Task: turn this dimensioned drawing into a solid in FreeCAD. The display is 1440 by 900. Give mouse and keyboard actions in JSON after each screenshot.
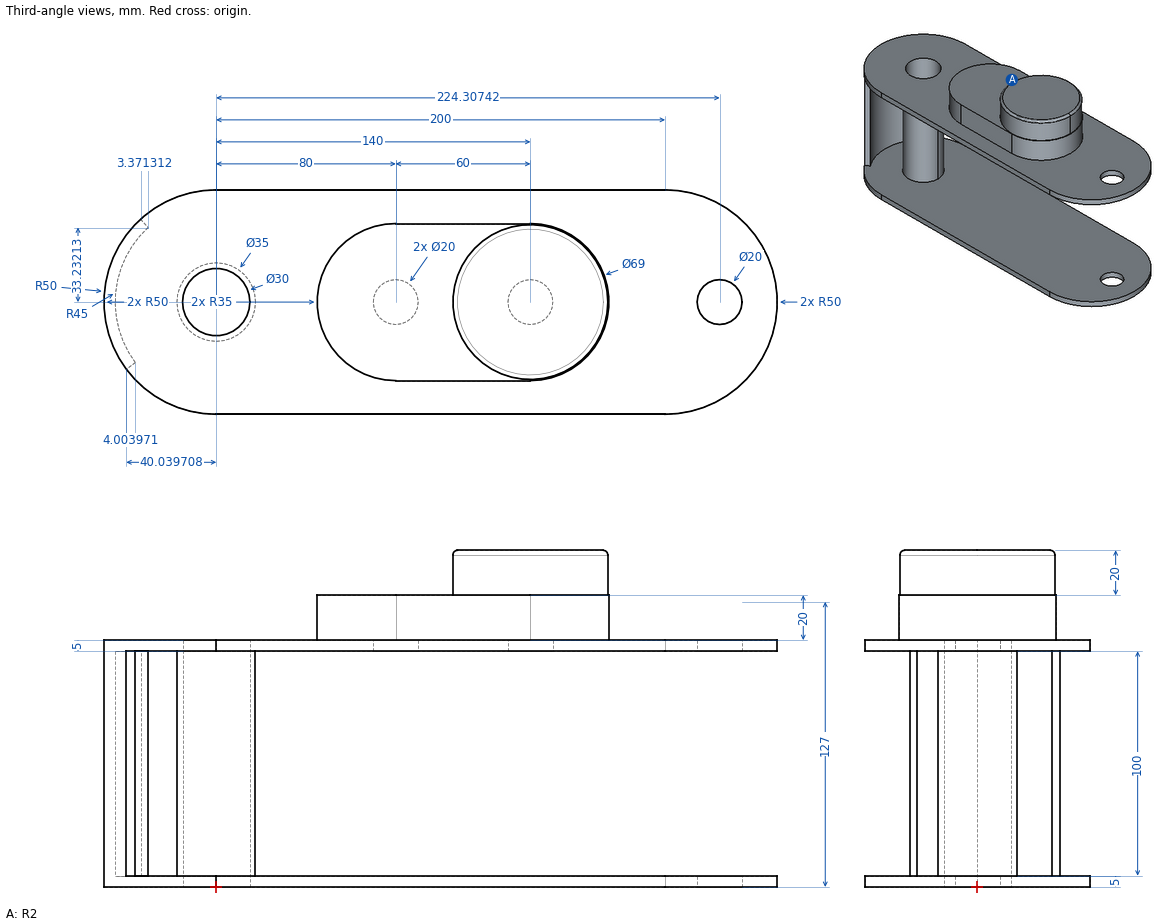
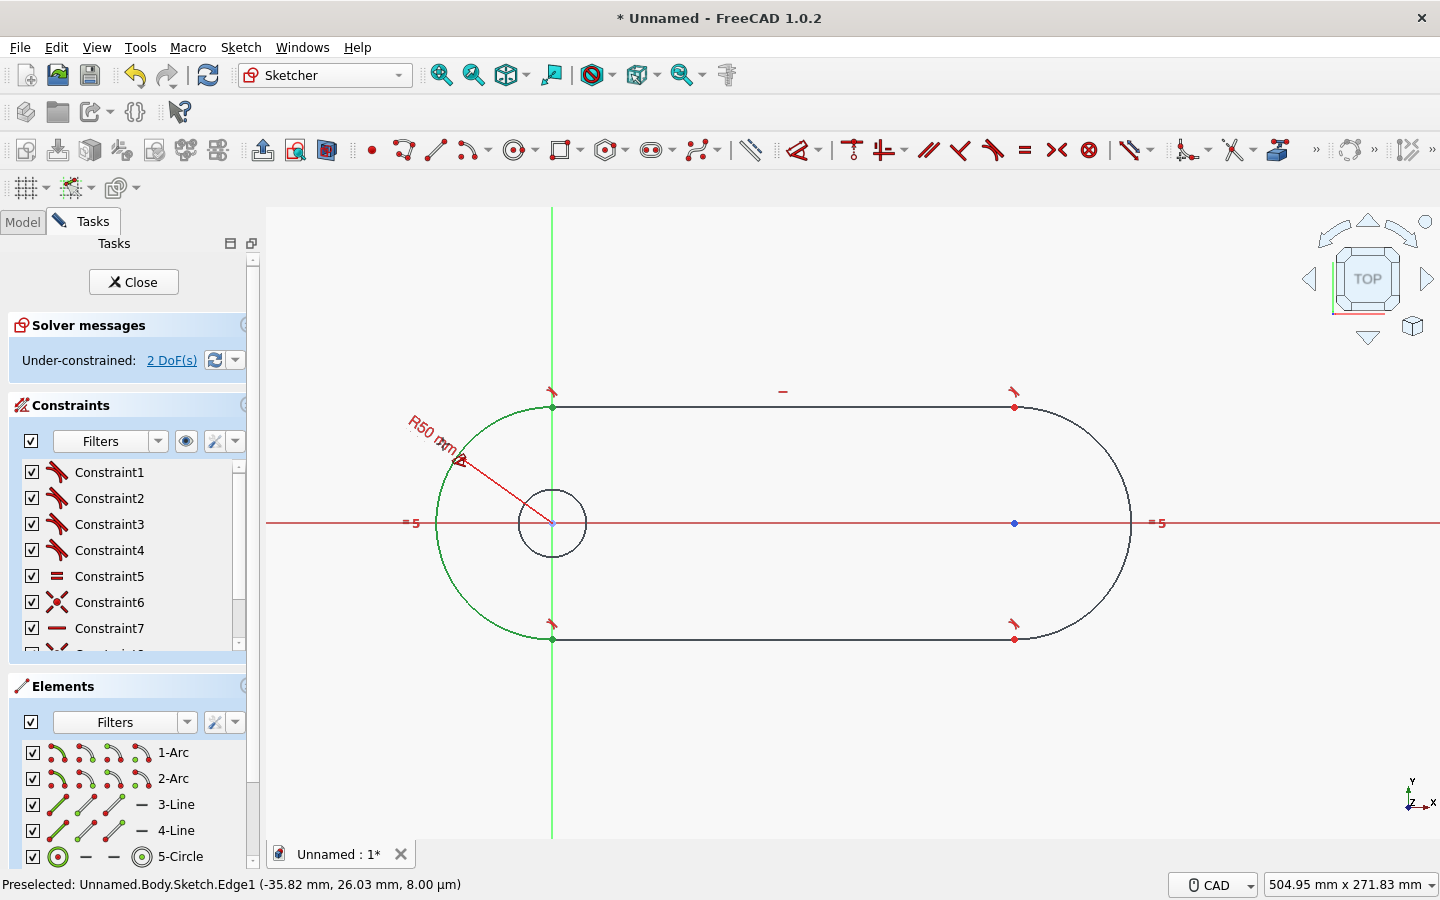
{"action": "left_click", "coordinate": [576, 499]}
{"action": "left_click", "coordinate": [598, 476]}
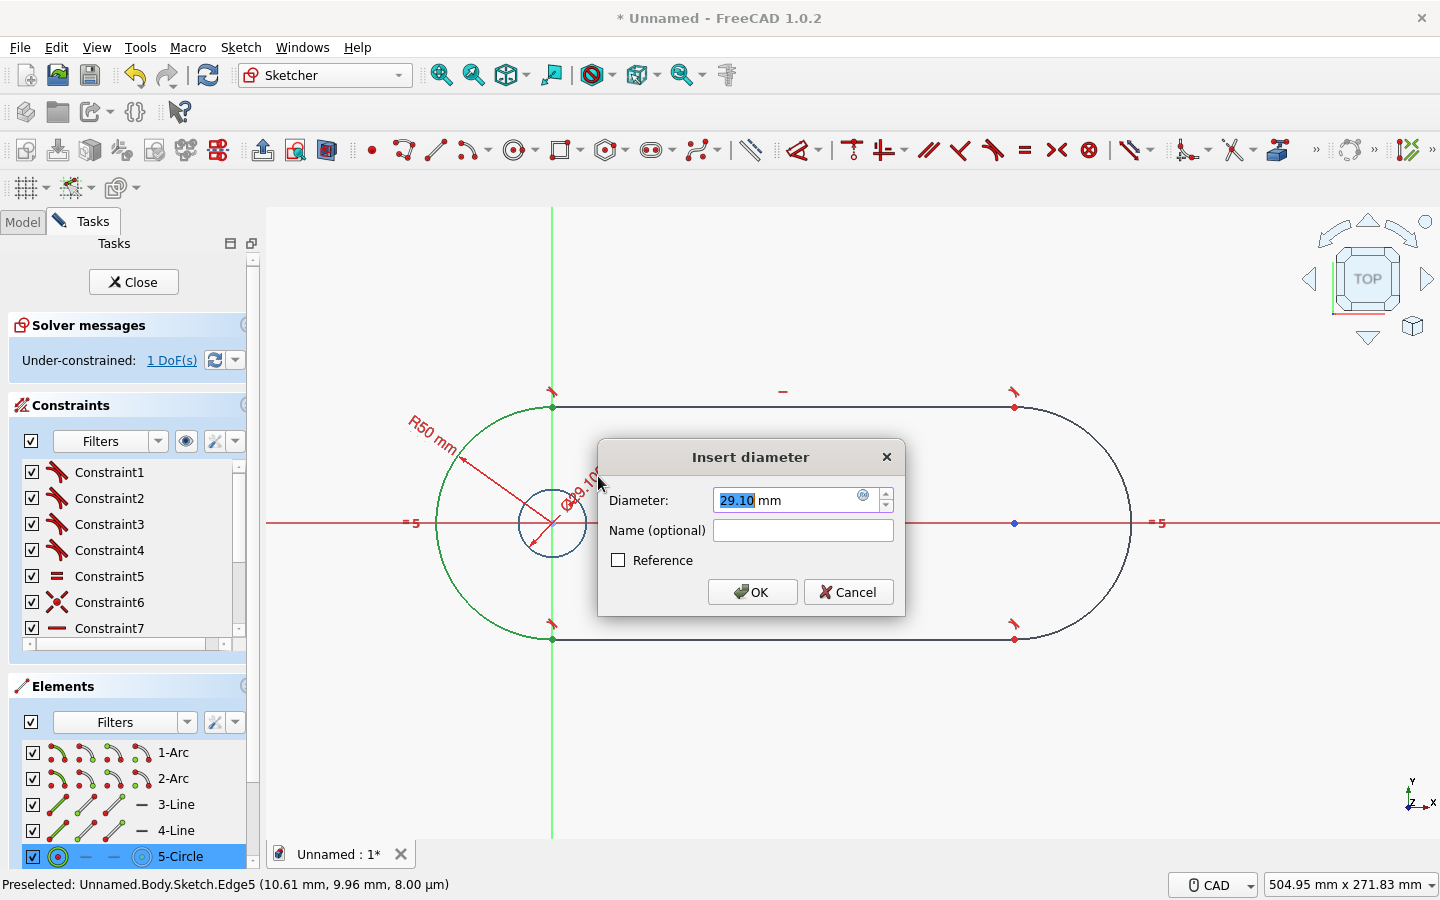
{"action": "type", "text": "30"}
{"action": "key", "text": "Return"}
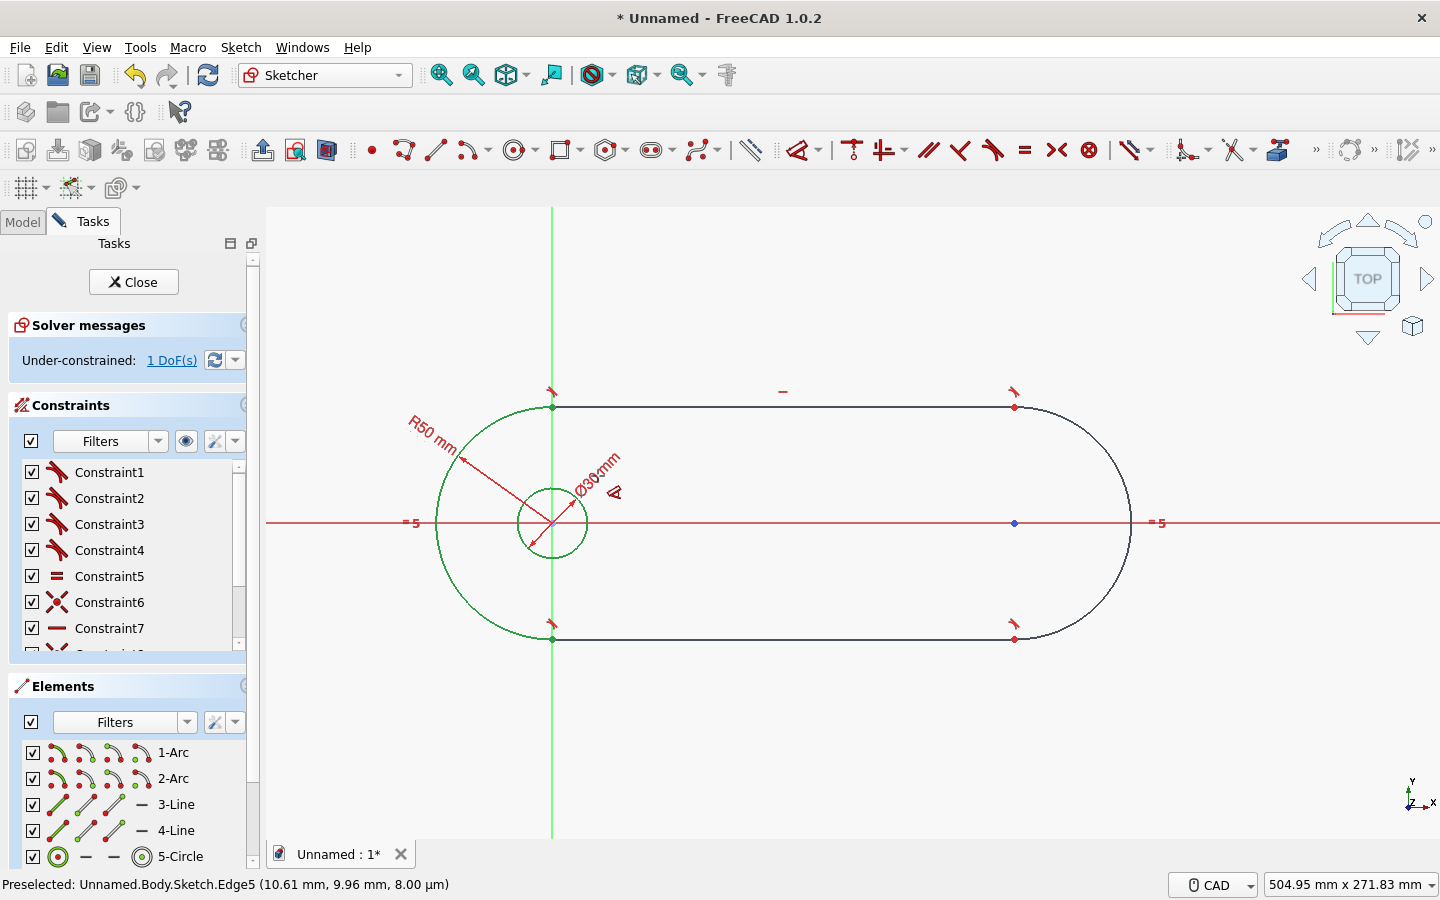
{"action": "left_click", "coordinate": [691, 407]}
{"action": "left_click", "coordinate": [784, 373]}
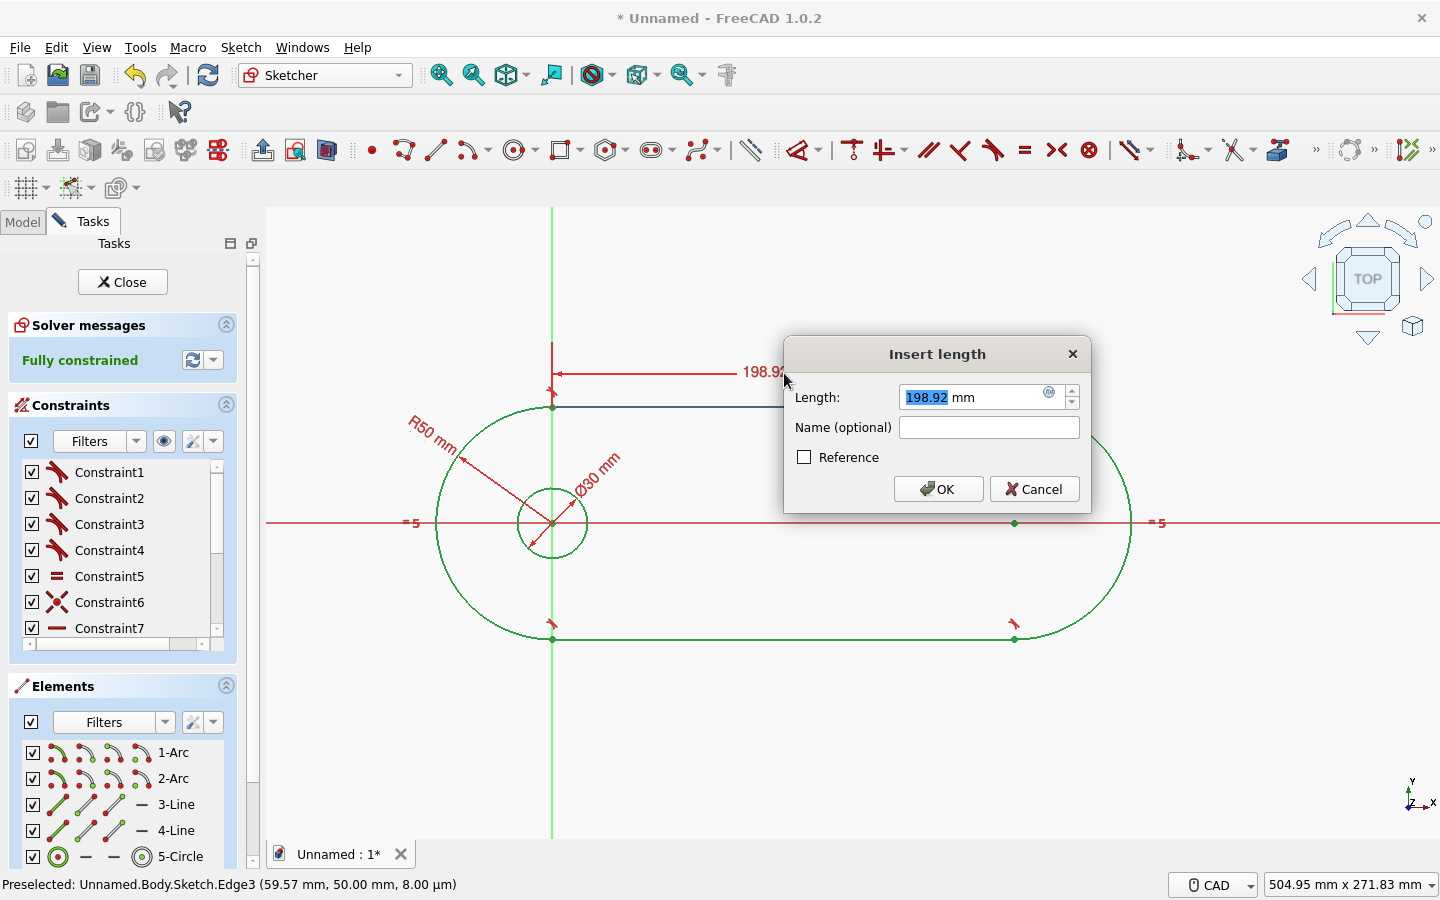
{"action": "type", "text": "200"}
{"action": "key", "text": "Return"}
{"action": "key", "text": "Escape"}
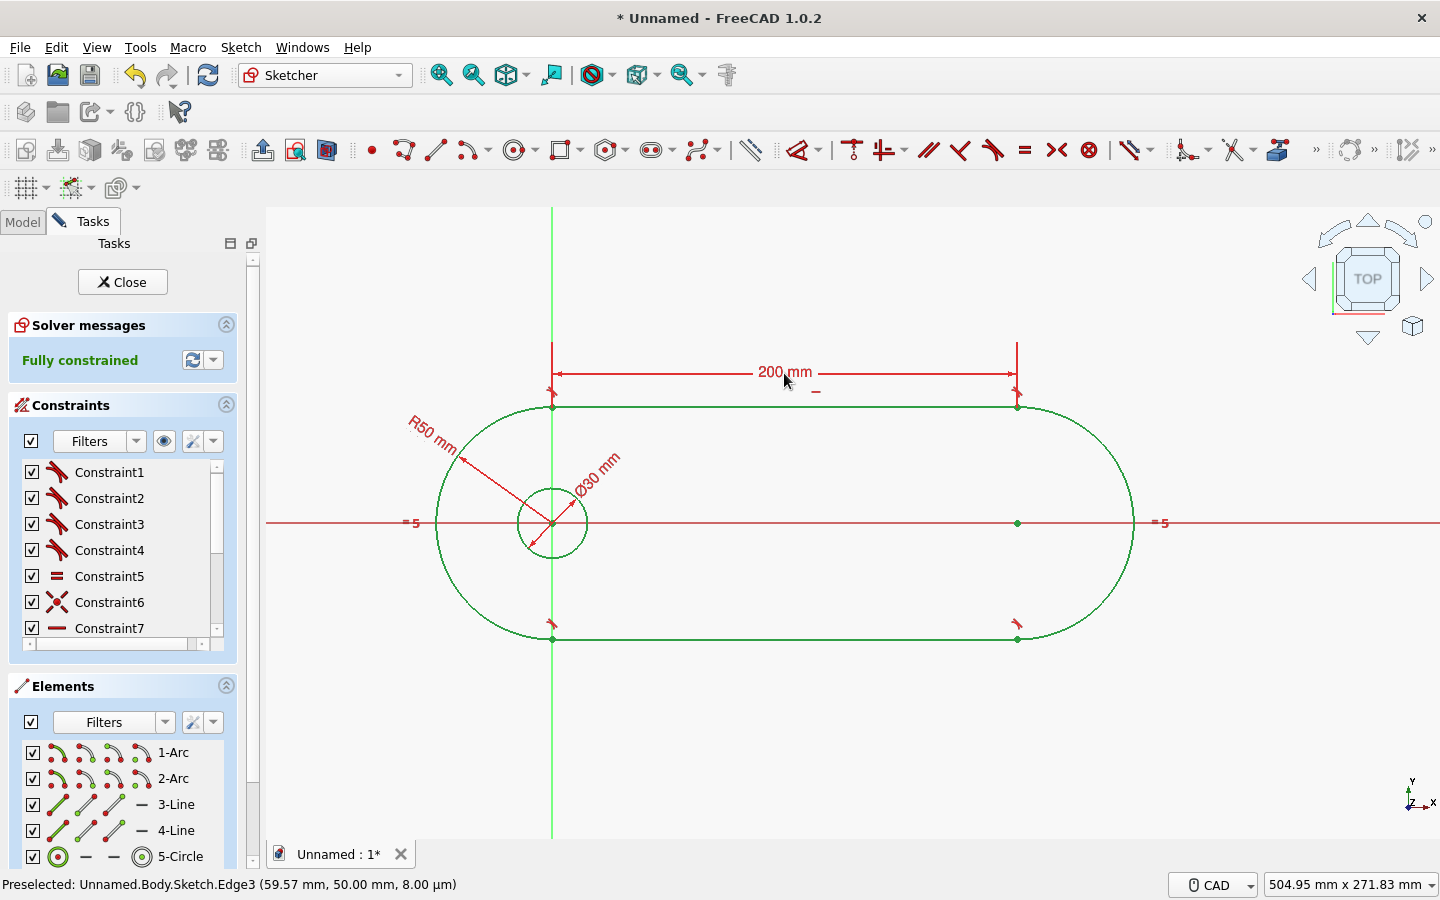
{"action": "left_click", "coordinate": [123, 282]}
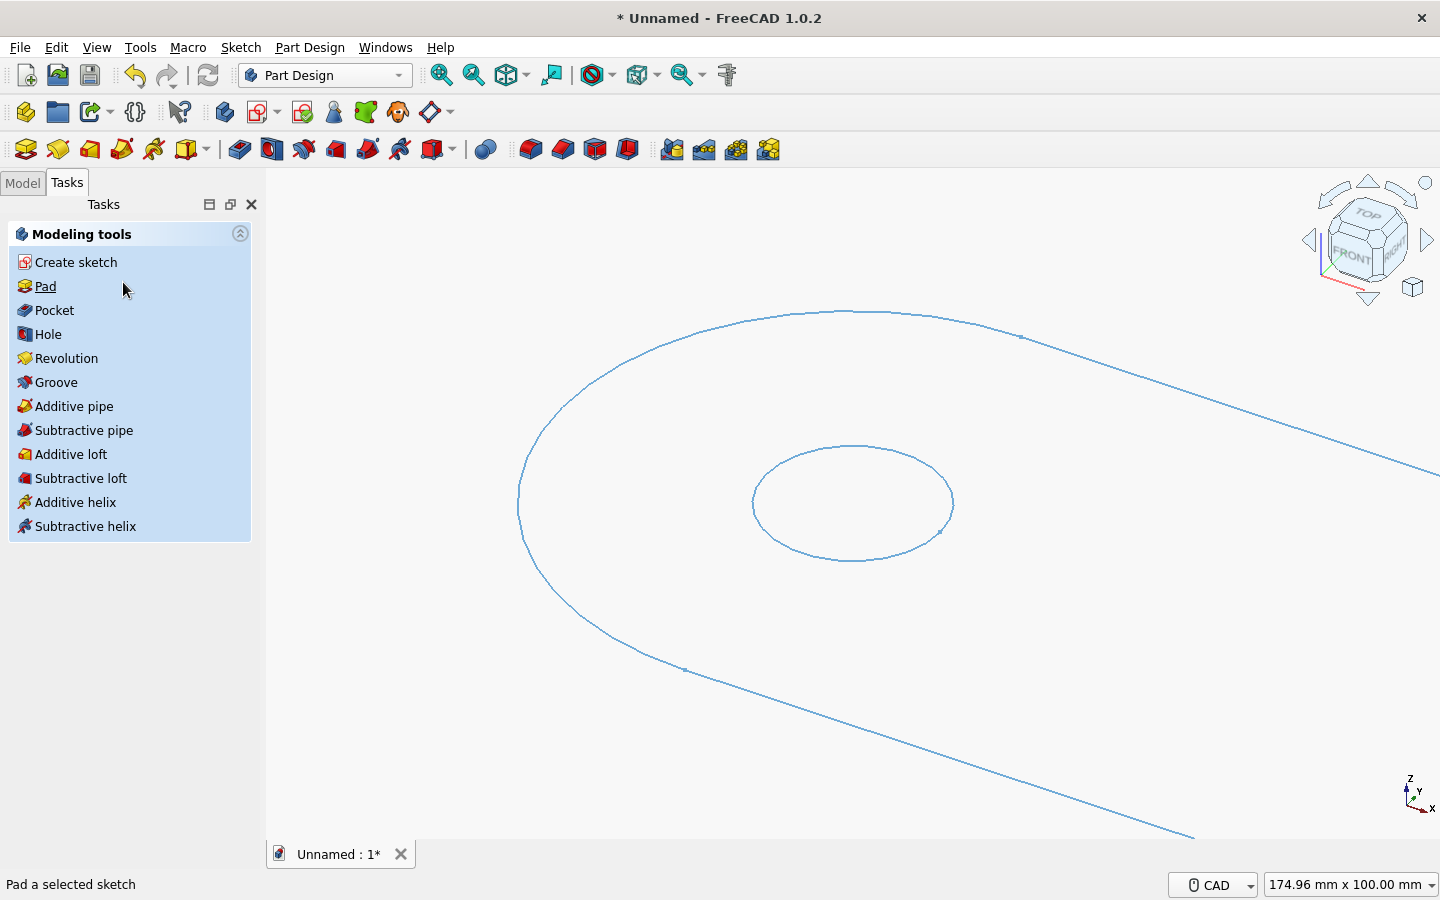
{"action": "left_click", "coordinate": [26, 150]}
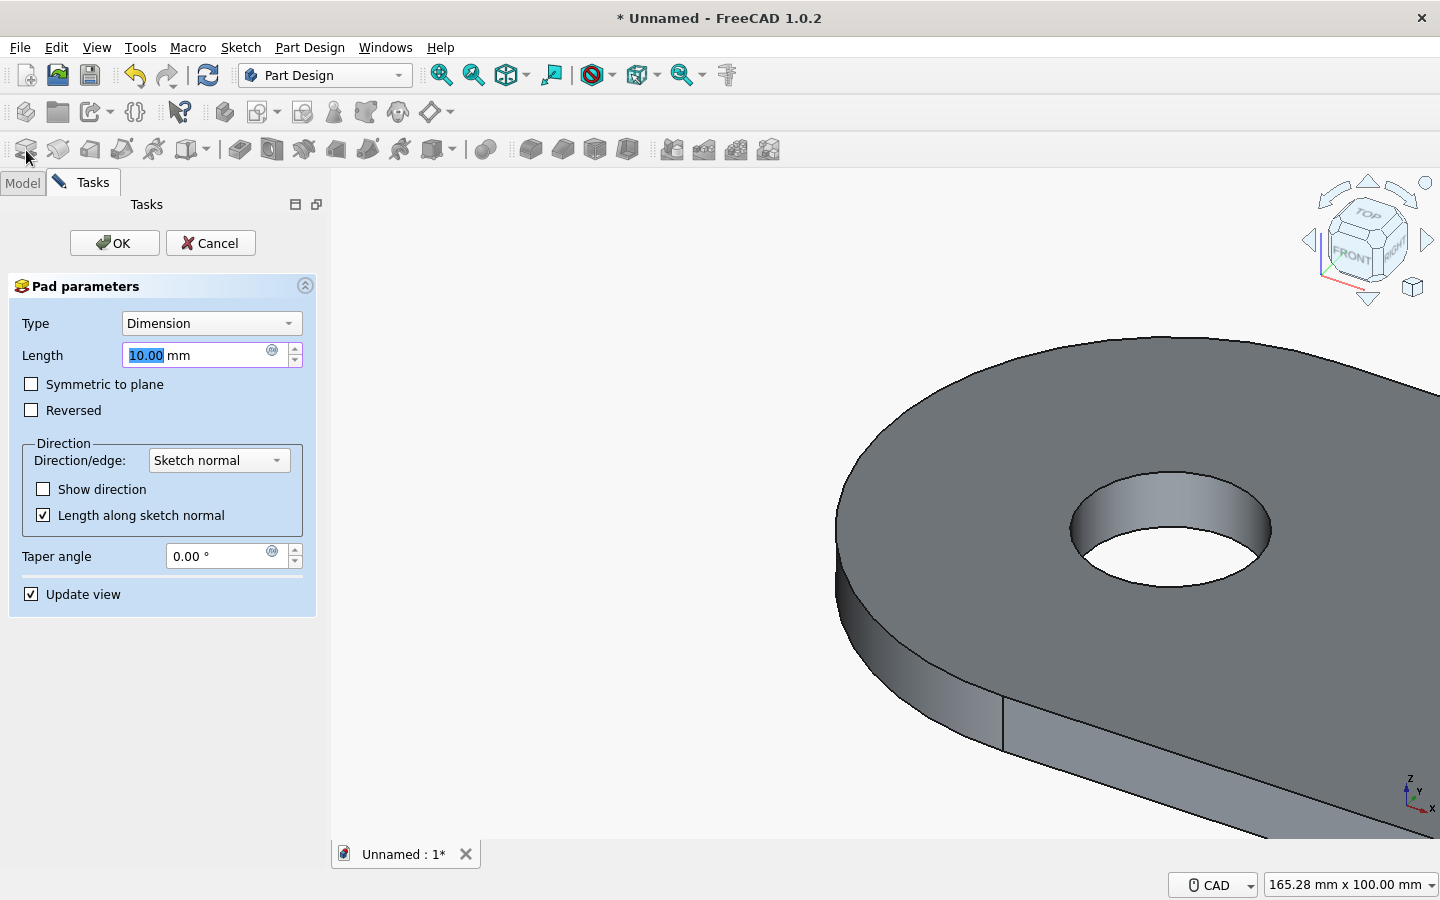
{"action": "type", "text": "5"}
{"action": "key", "text": "Tab"}